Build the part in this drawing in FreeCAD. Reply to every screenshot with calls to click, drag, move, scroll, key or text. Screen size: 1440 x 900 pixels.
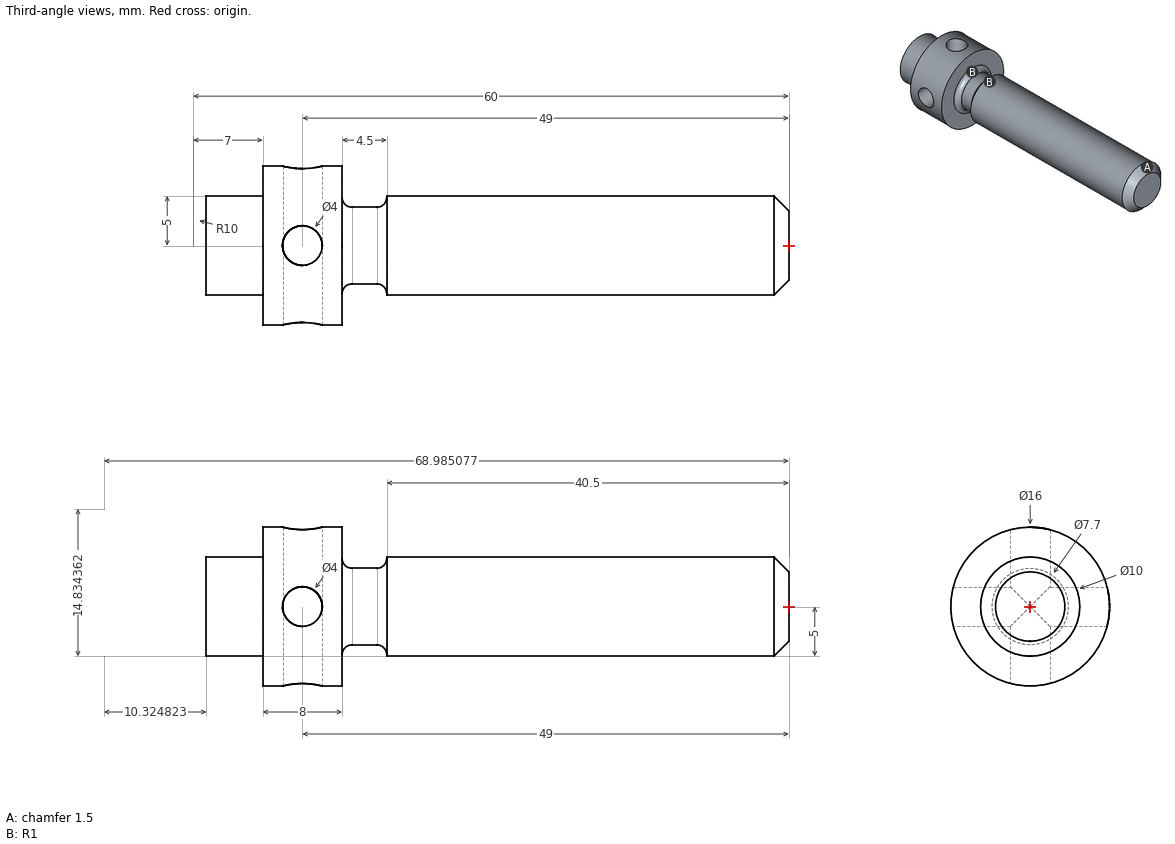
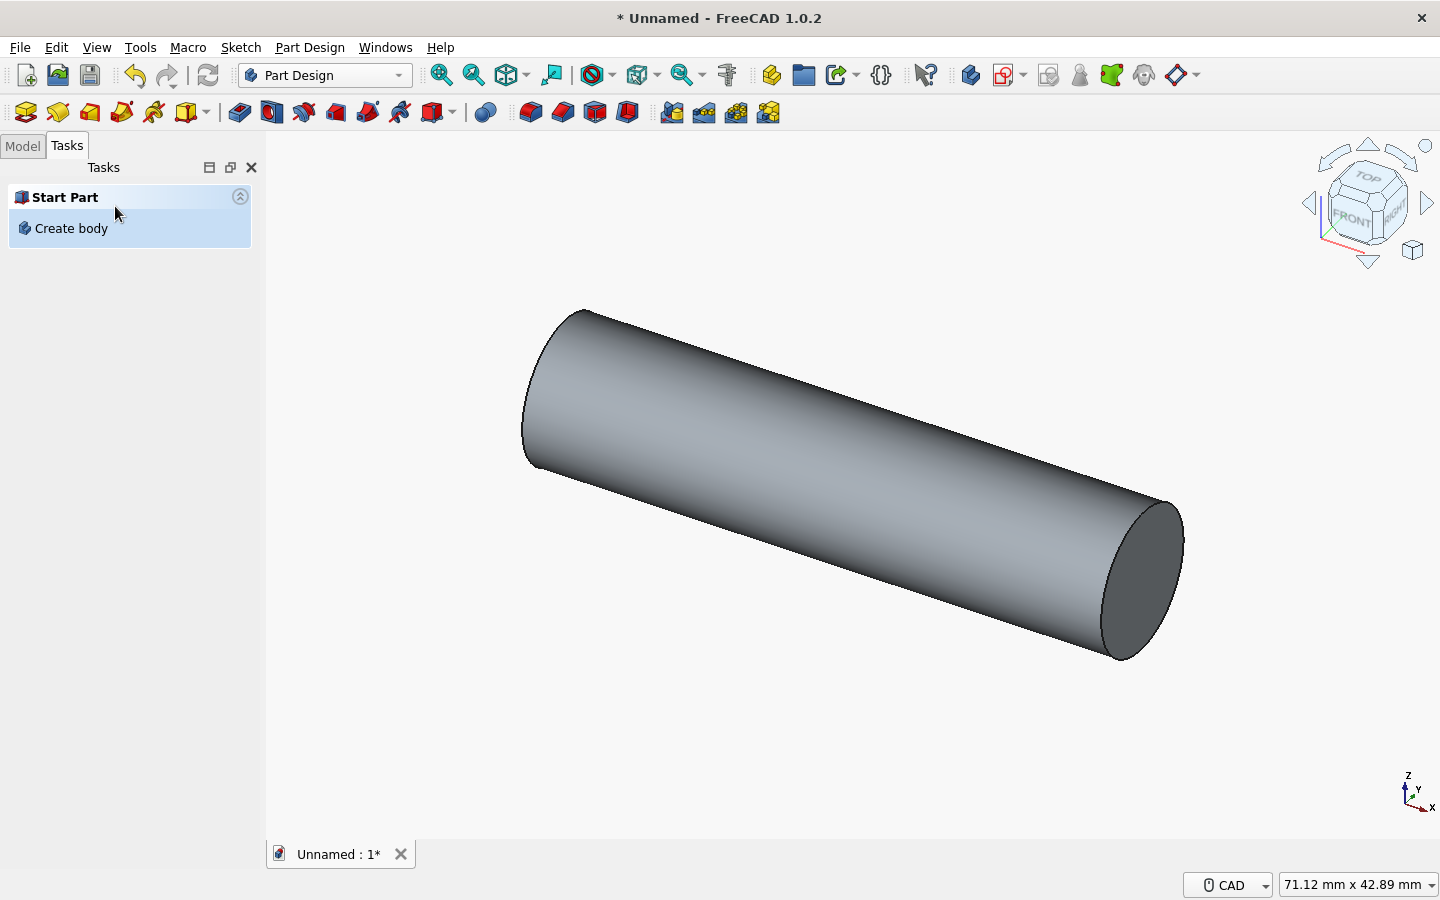
click(1101, 621)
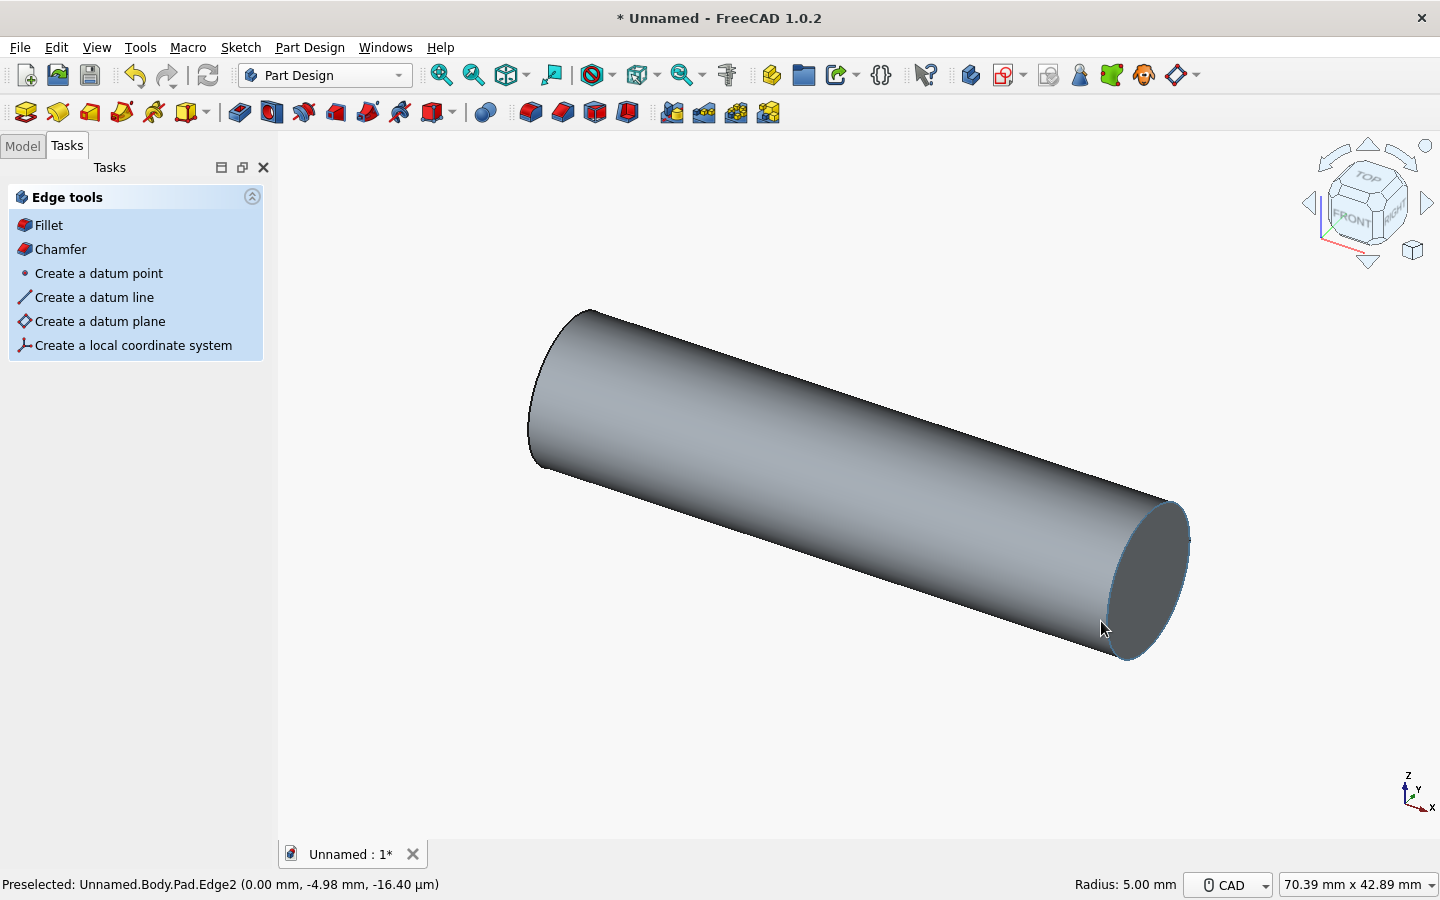
click(564, 112)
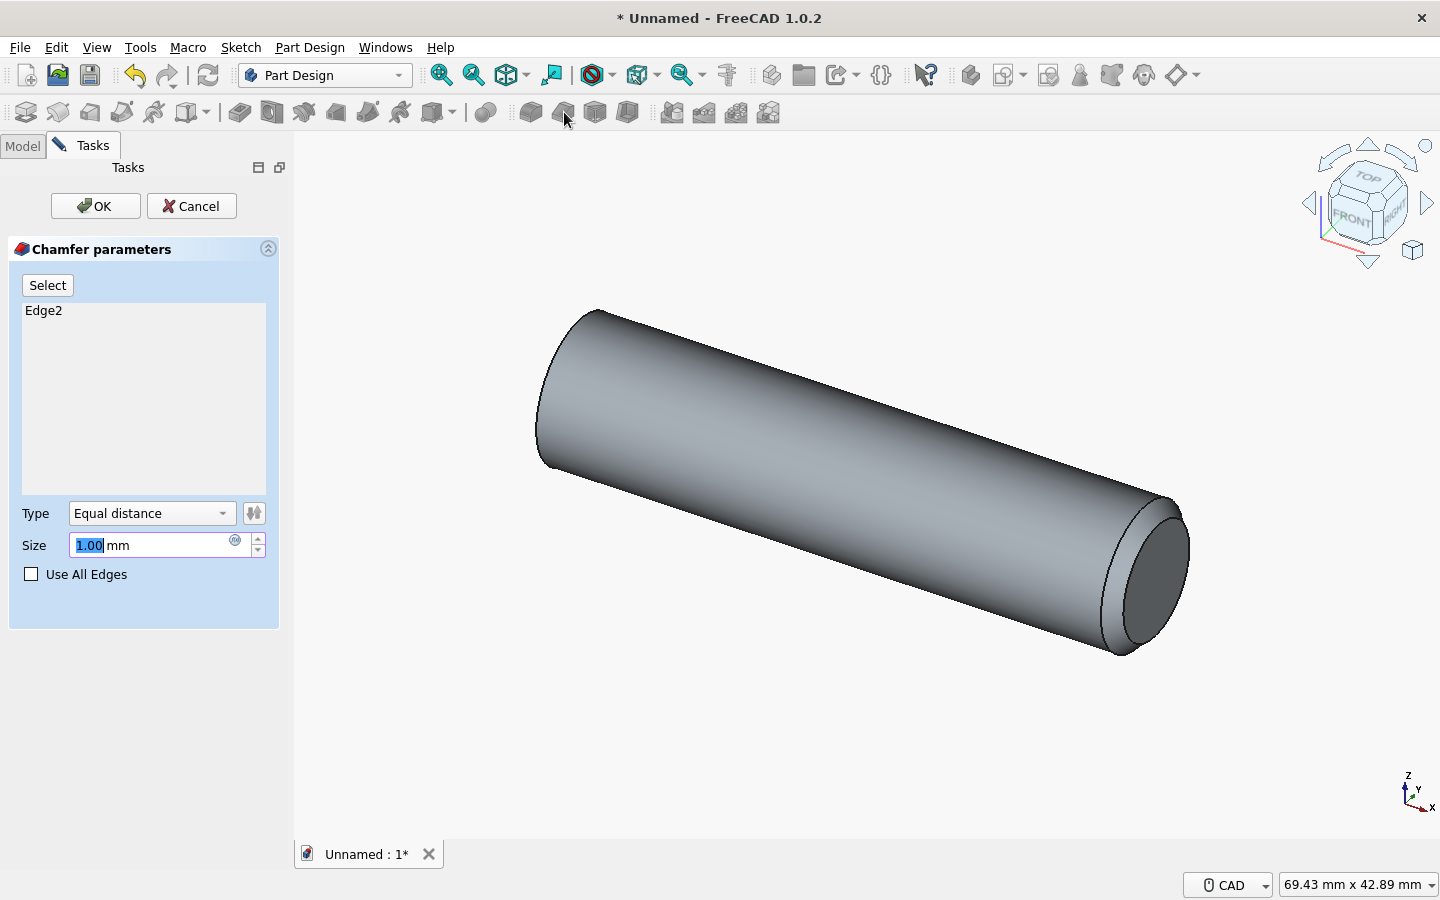
text(1.5)
key(Tab)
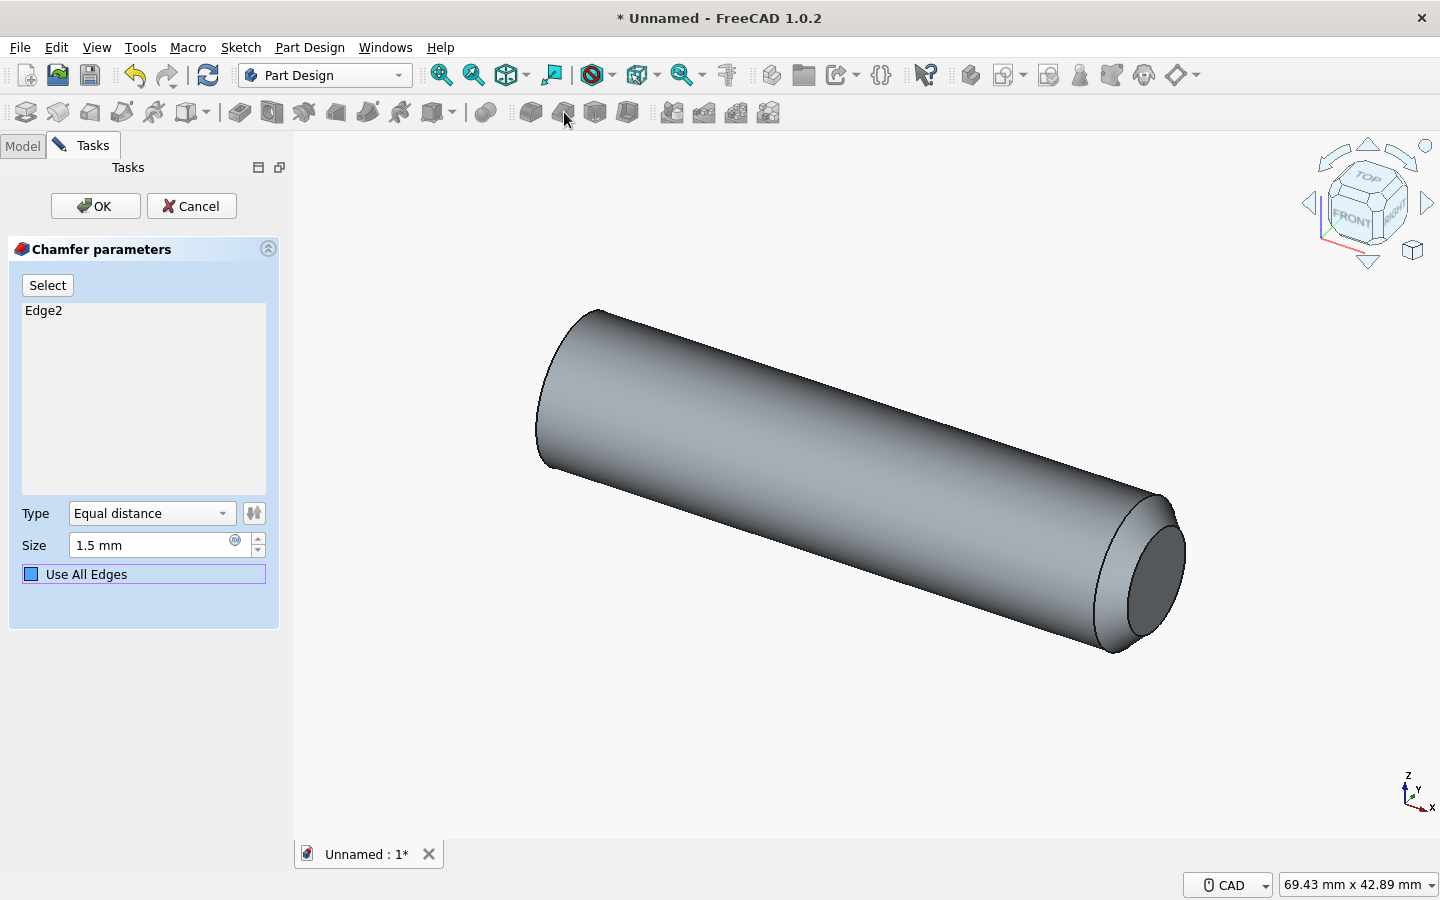
click(96, 206)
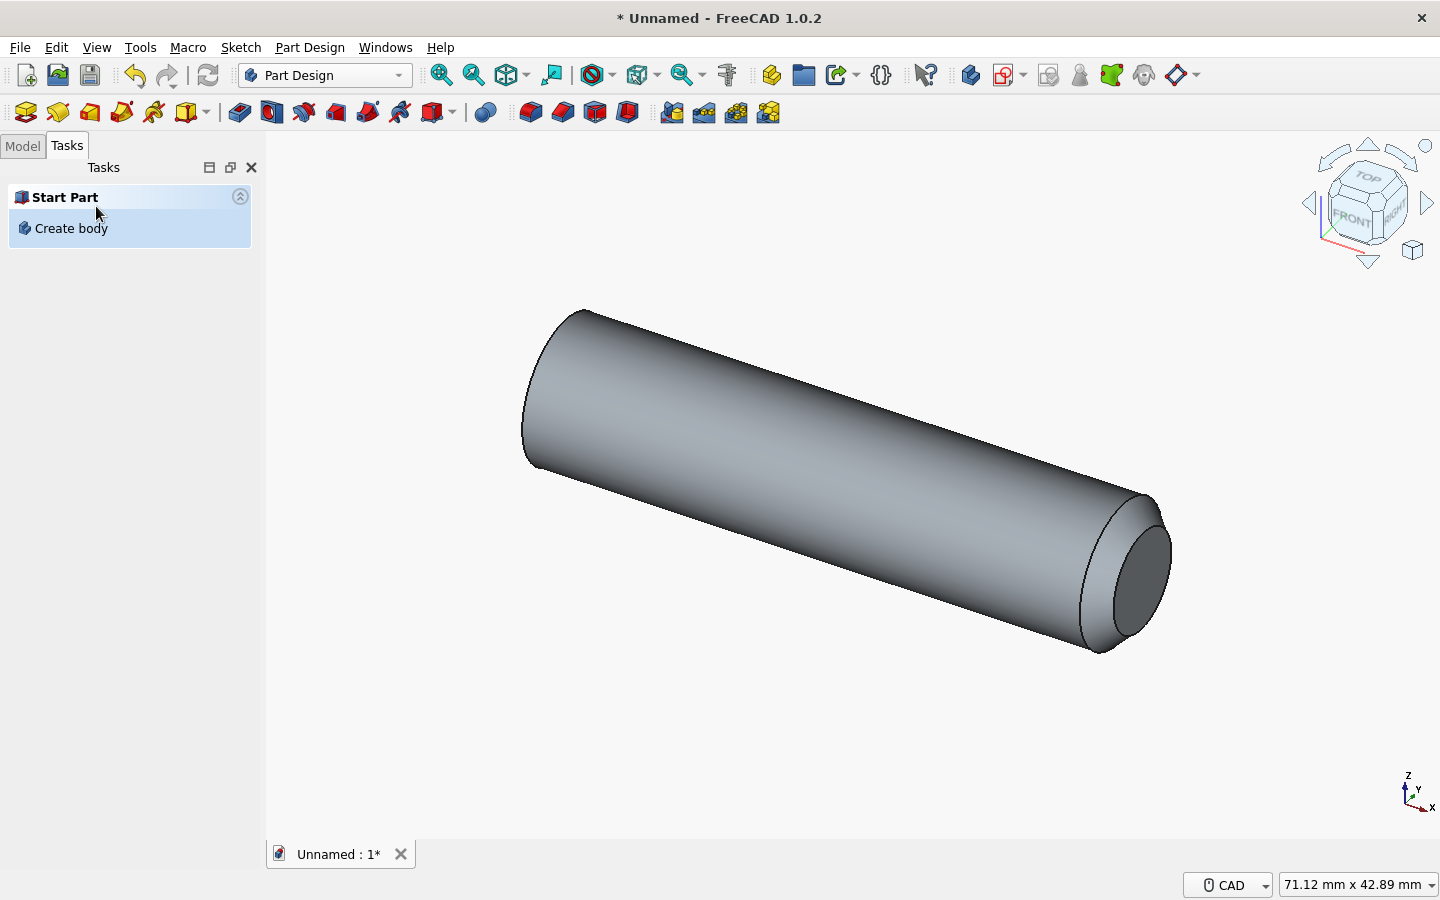
key(6)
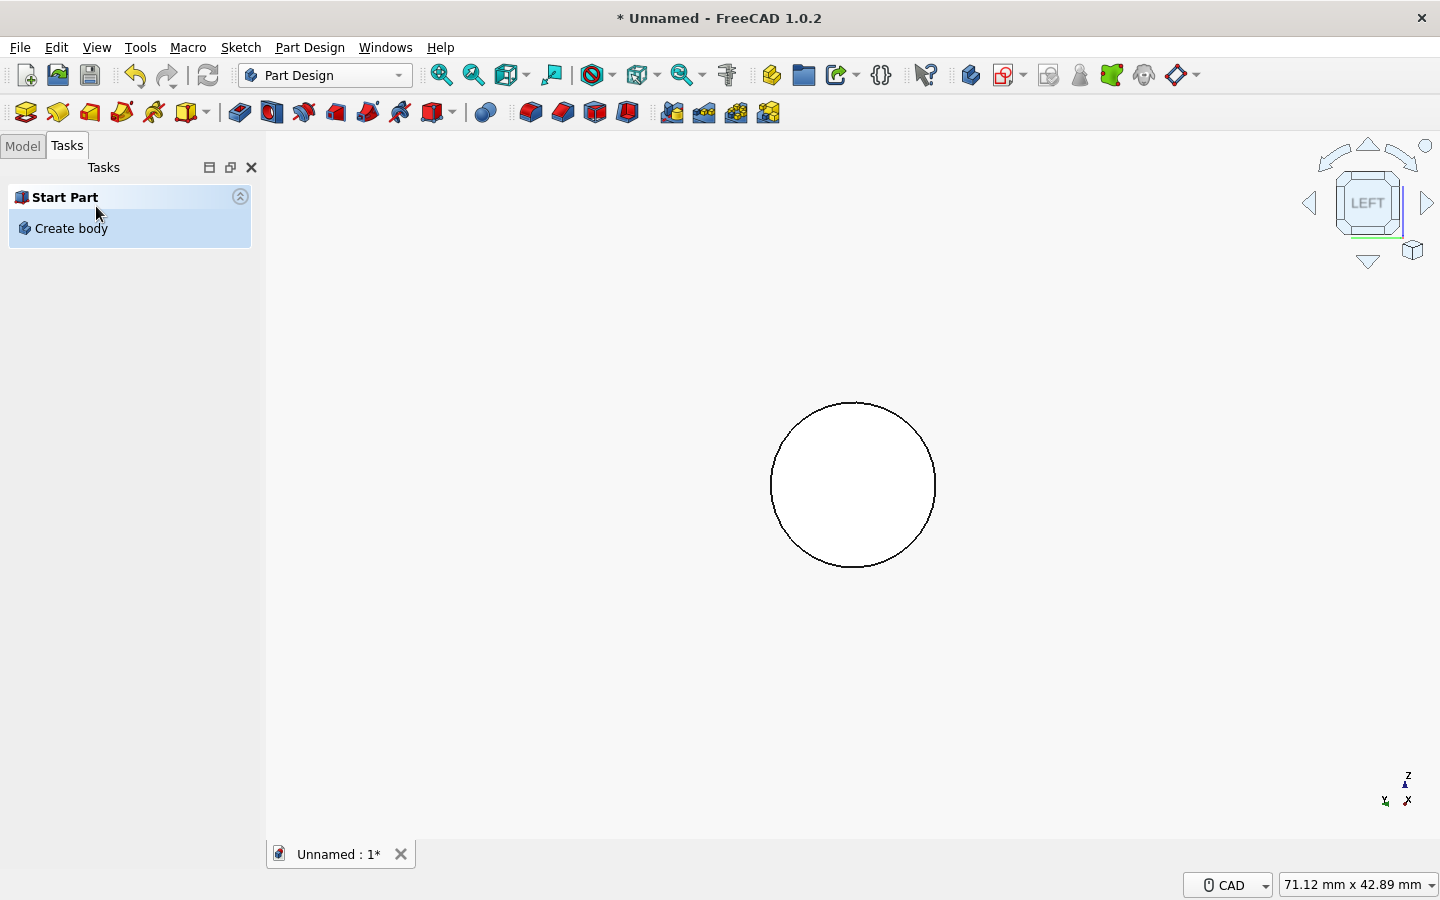
key(v)
key(f)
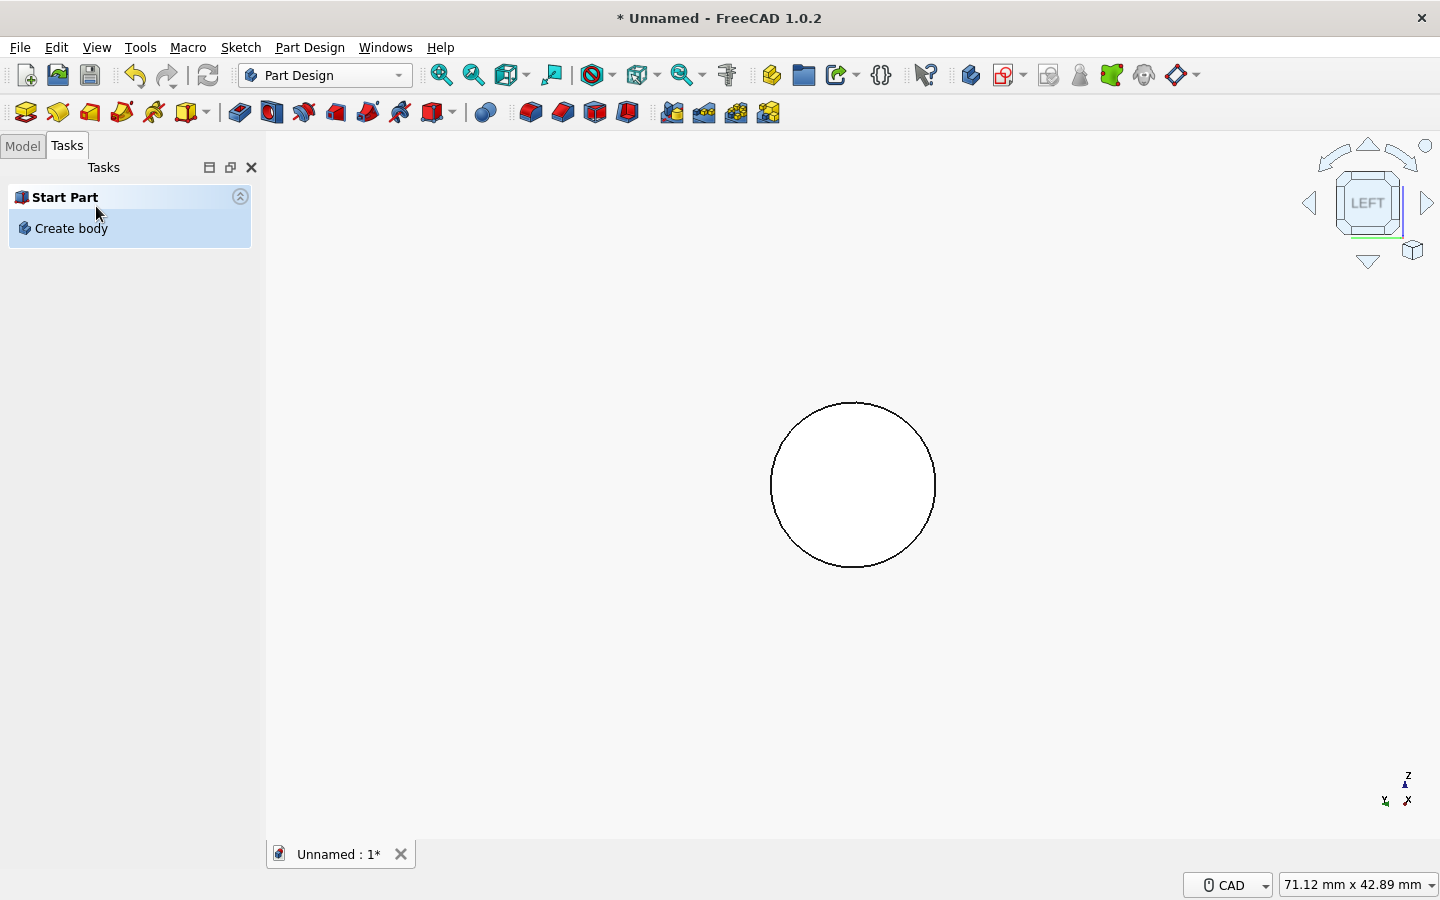
click(853, 484)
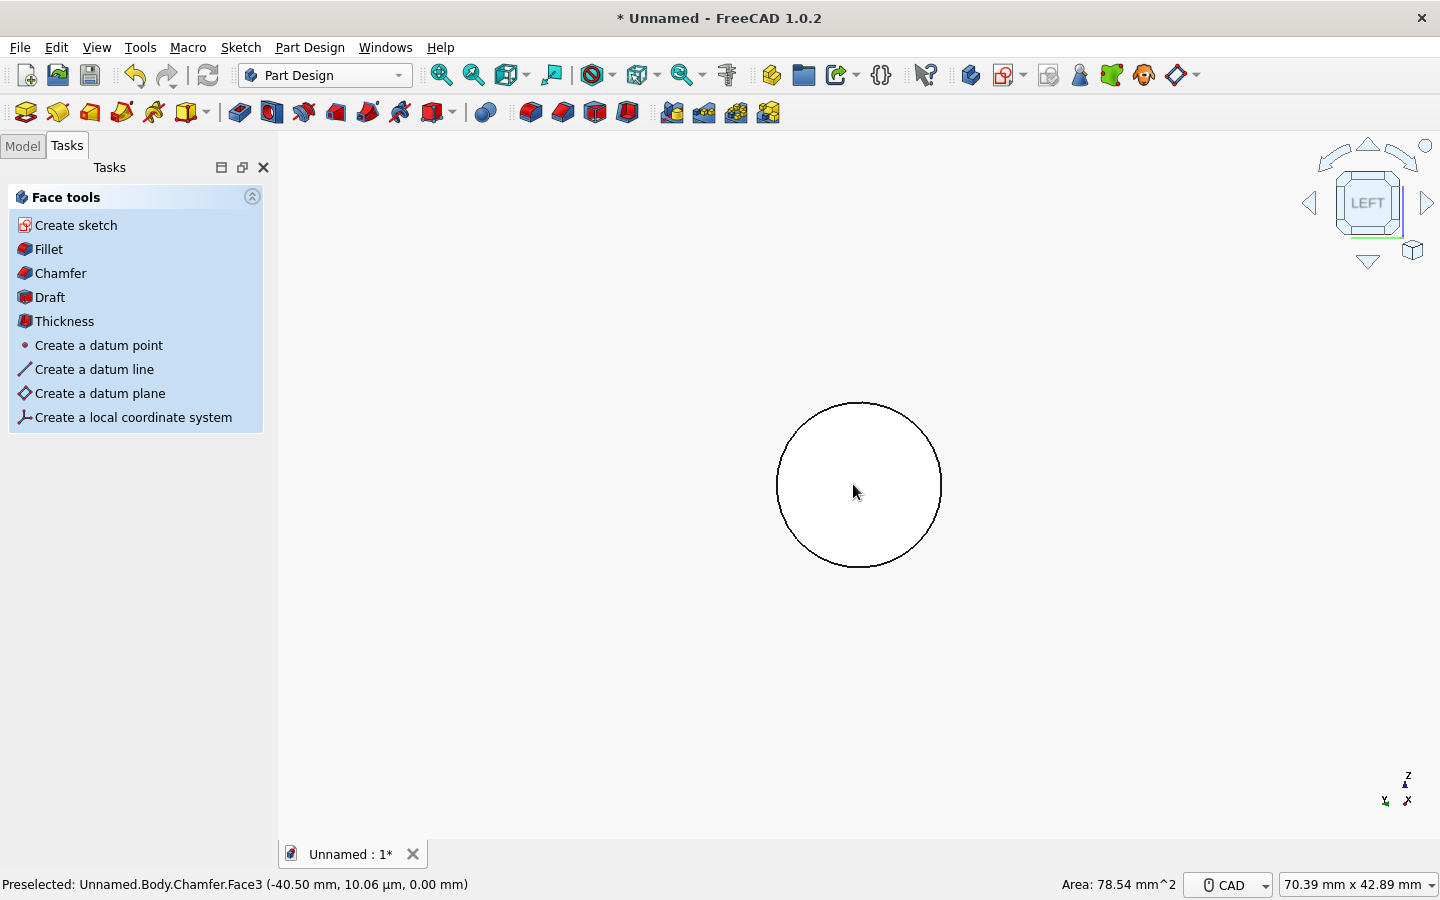
click(1004, 76)